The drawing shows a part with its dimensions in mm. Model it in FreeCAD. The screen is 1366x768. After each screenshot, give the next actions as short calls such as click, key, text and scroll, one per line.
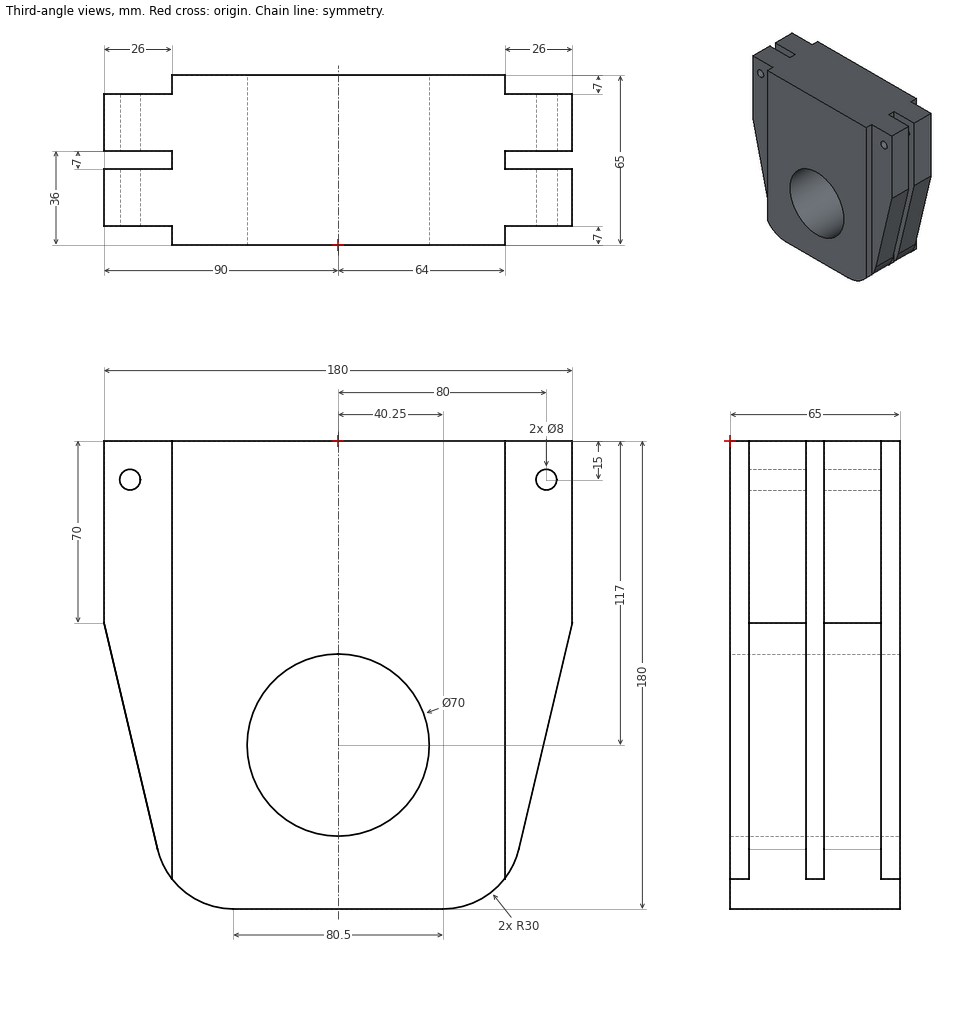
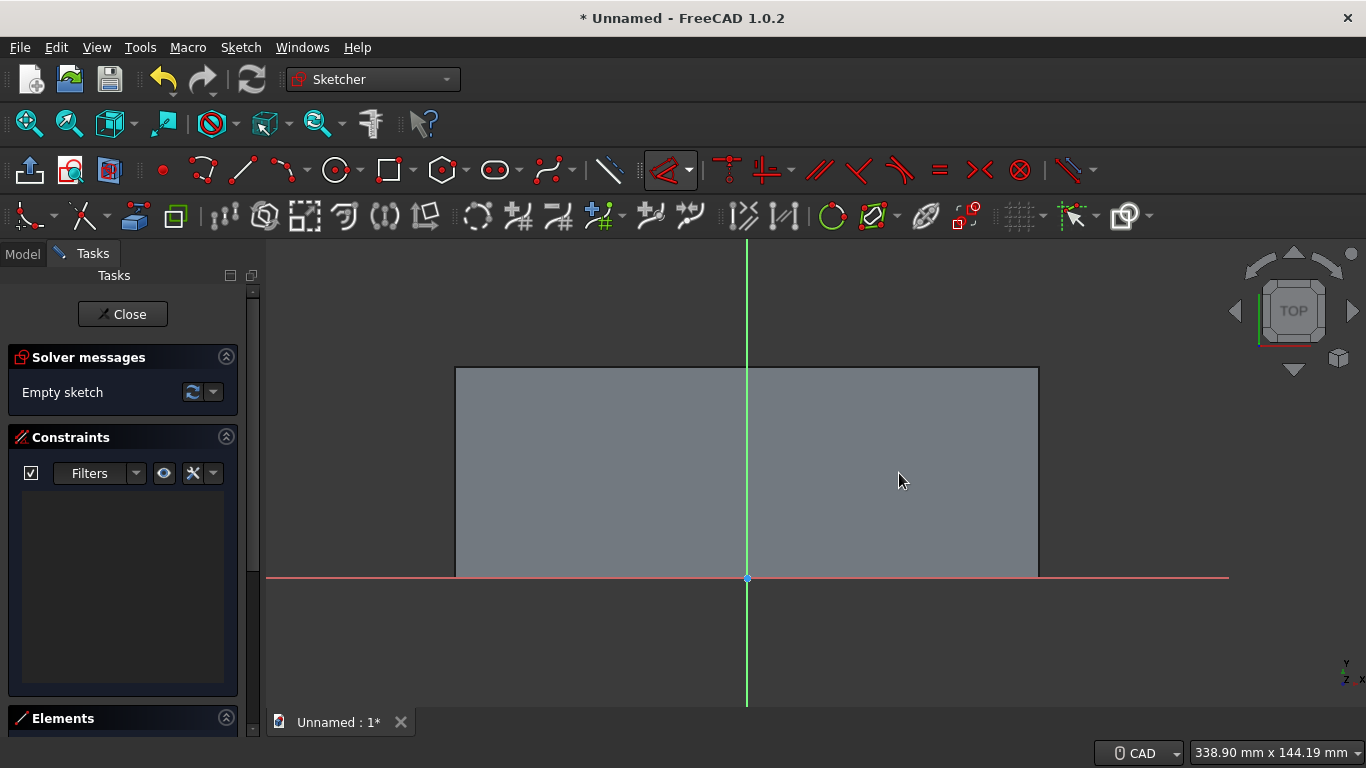
click(390, 170)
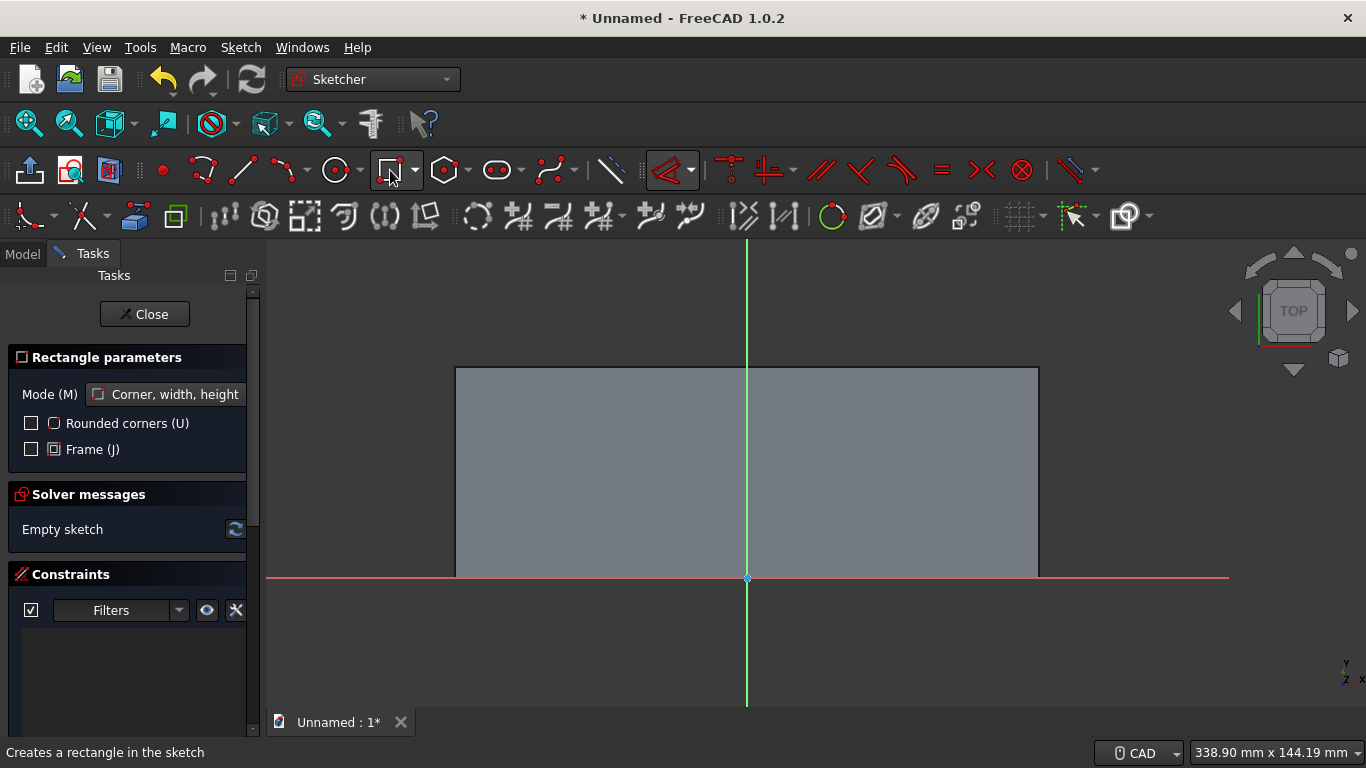
click(955, 555)
click(1039, 578)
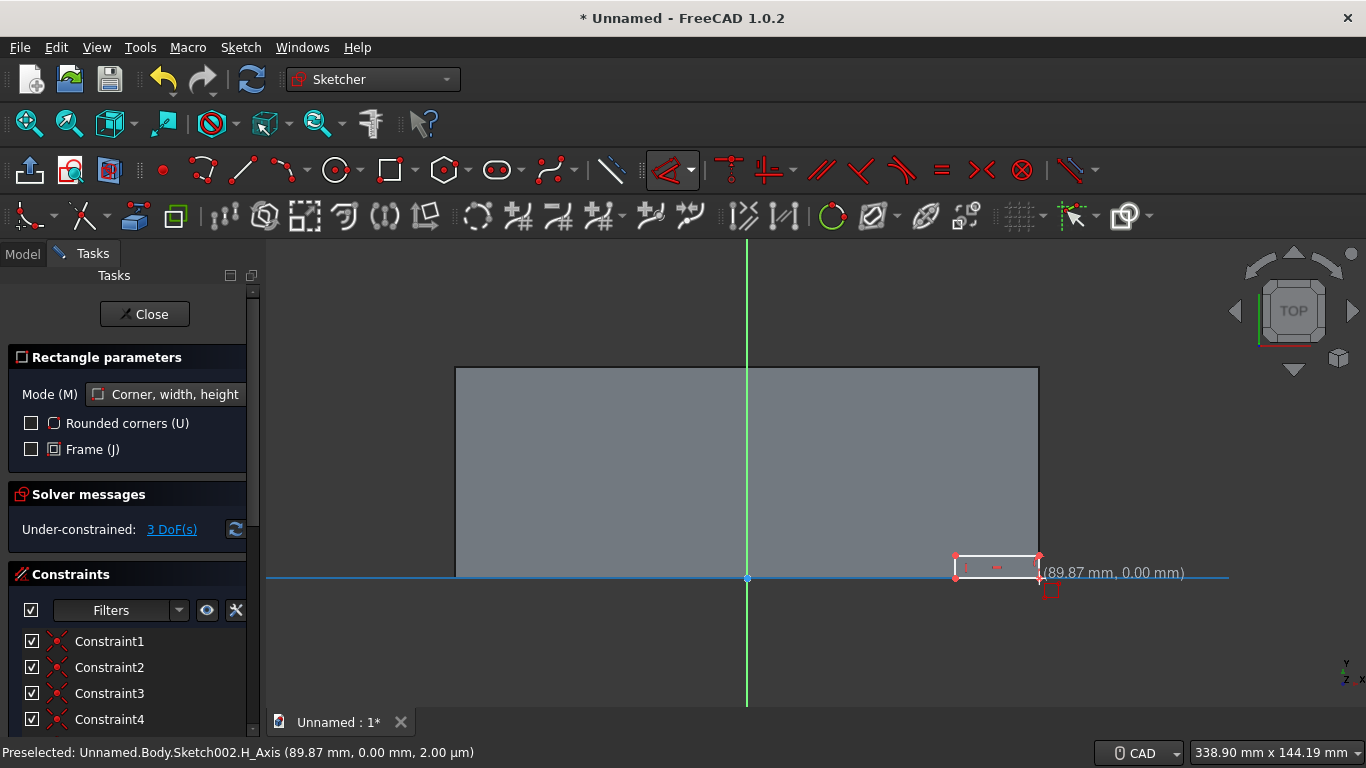
click(955, 367)
move(1039, 390)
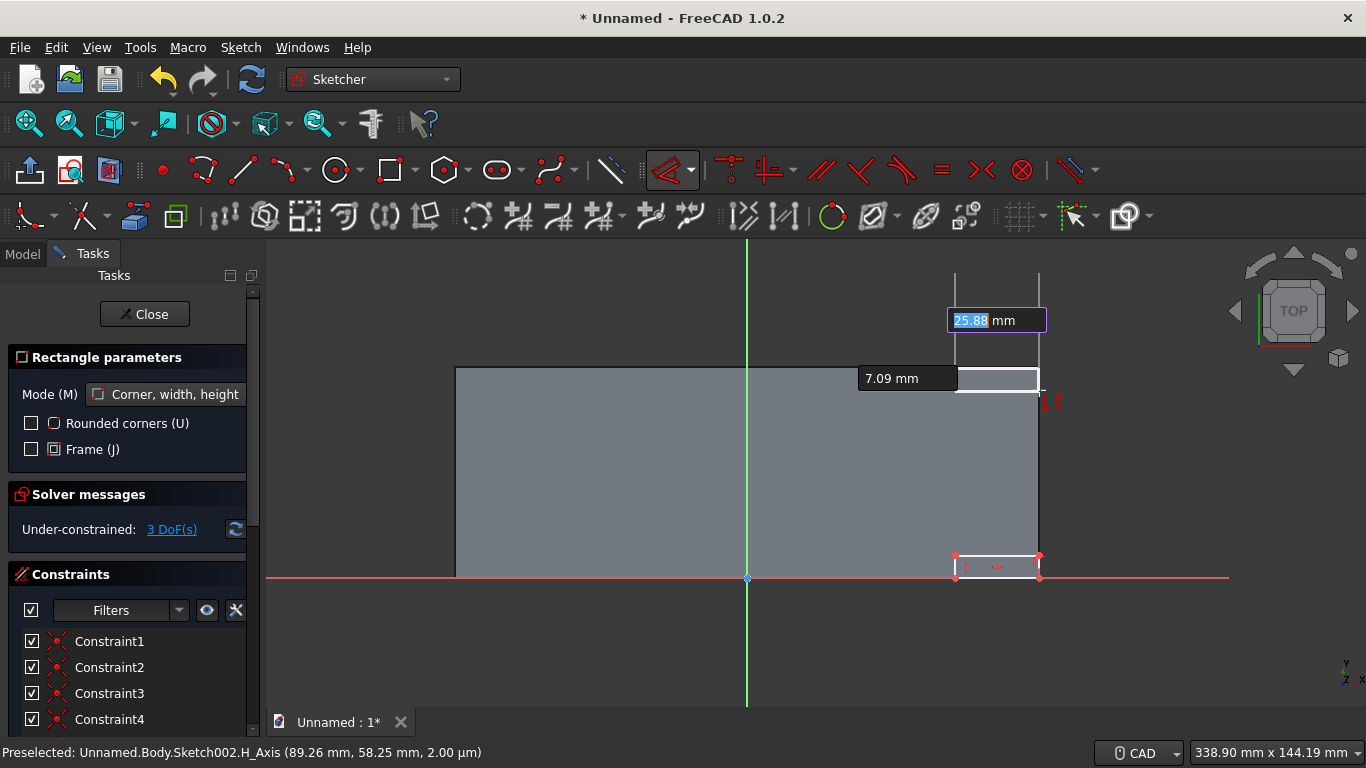
text(26)
key(Tab)
text(7)
key(Return)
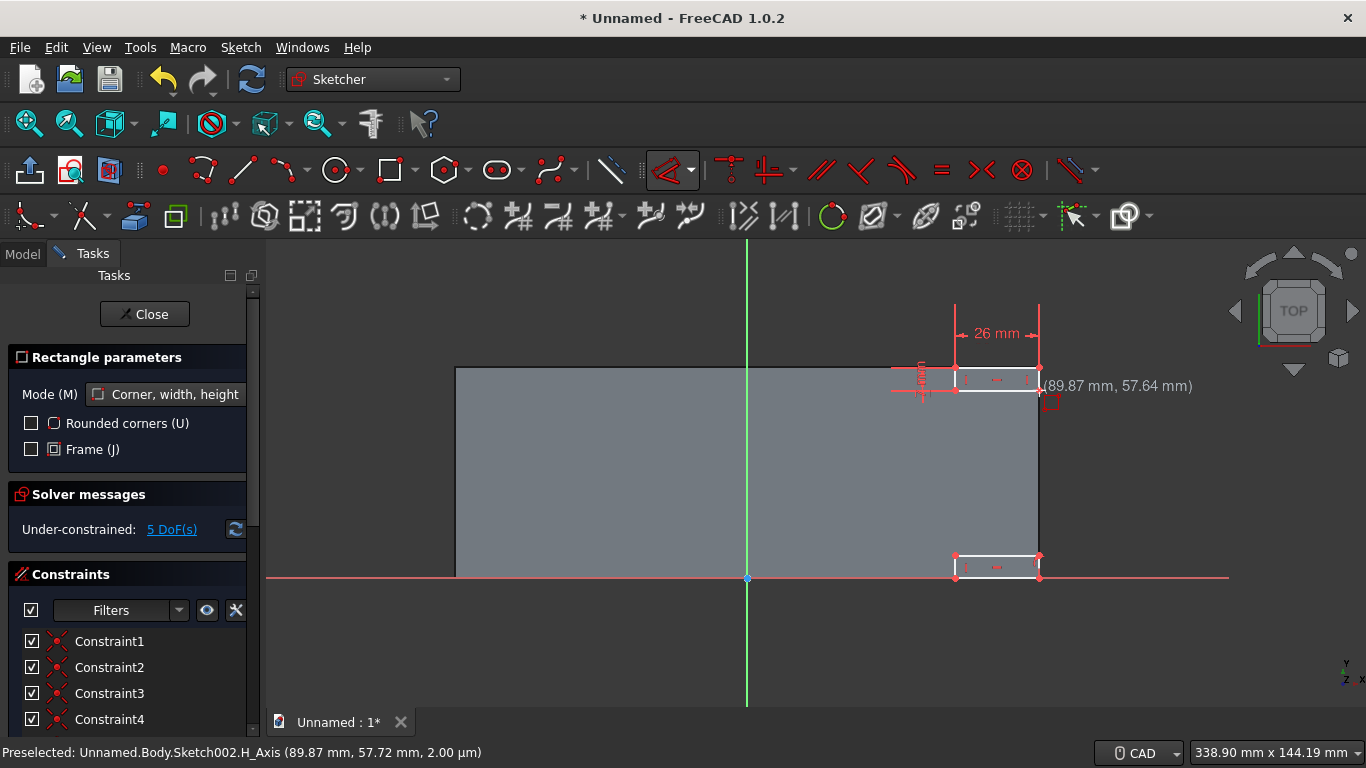
click(455, 367)
move(540, 390)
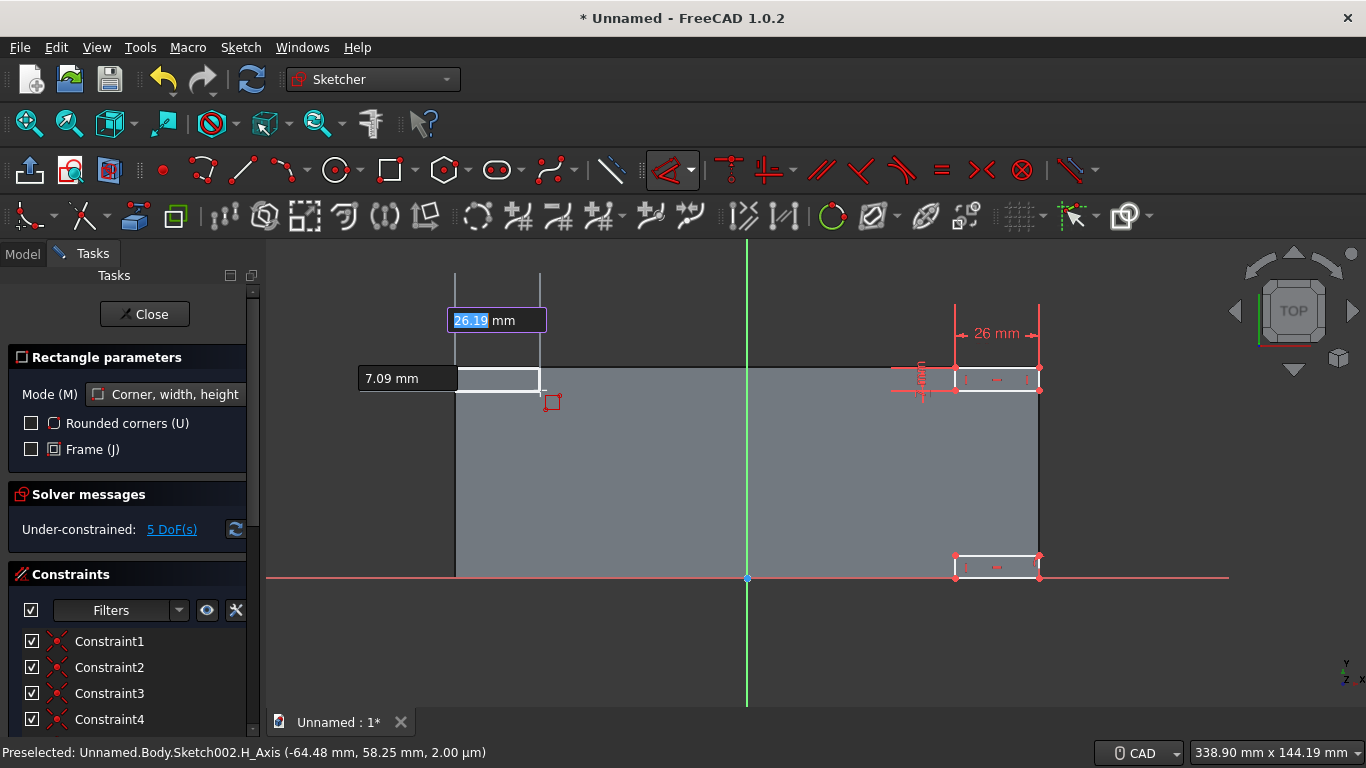
text(26)
key(Tab)
text(7)
key(Return)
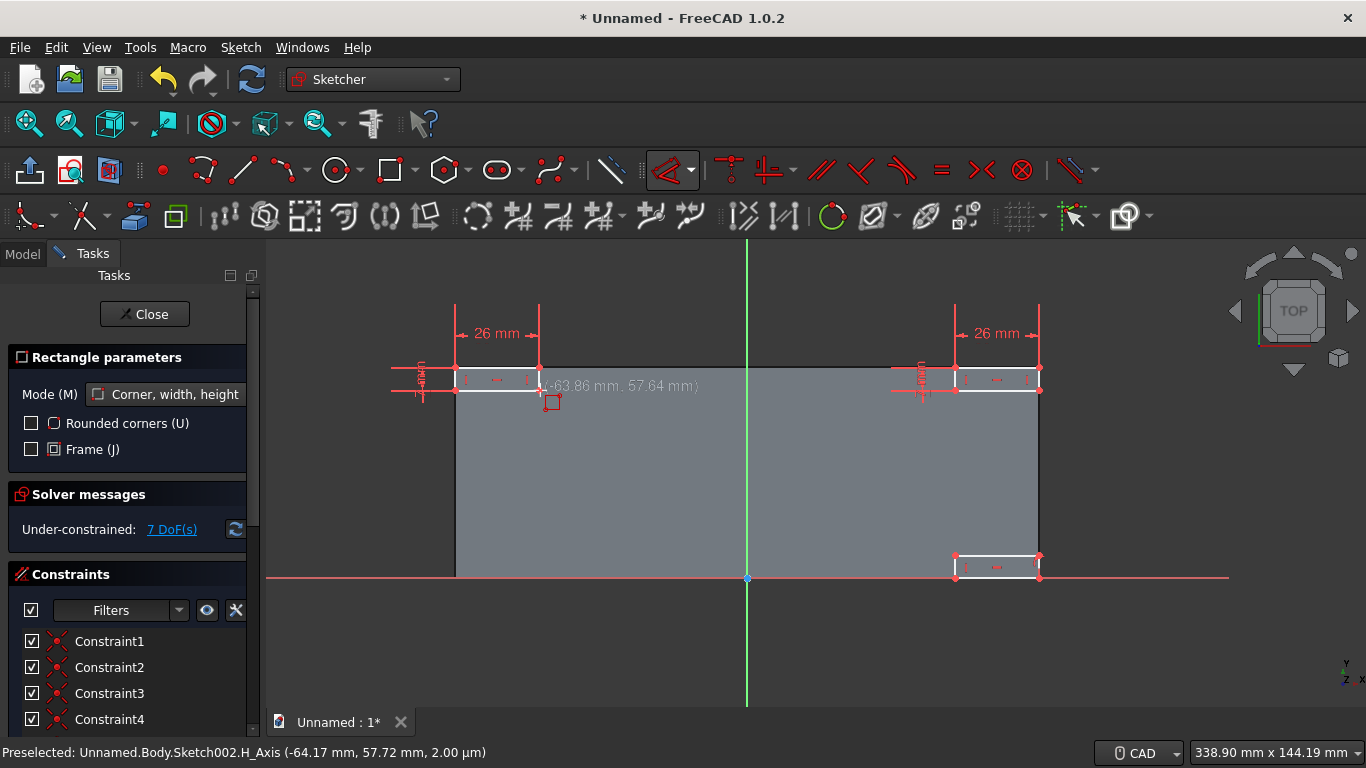
click(455, 555)
click(540, 578)
key(Escape)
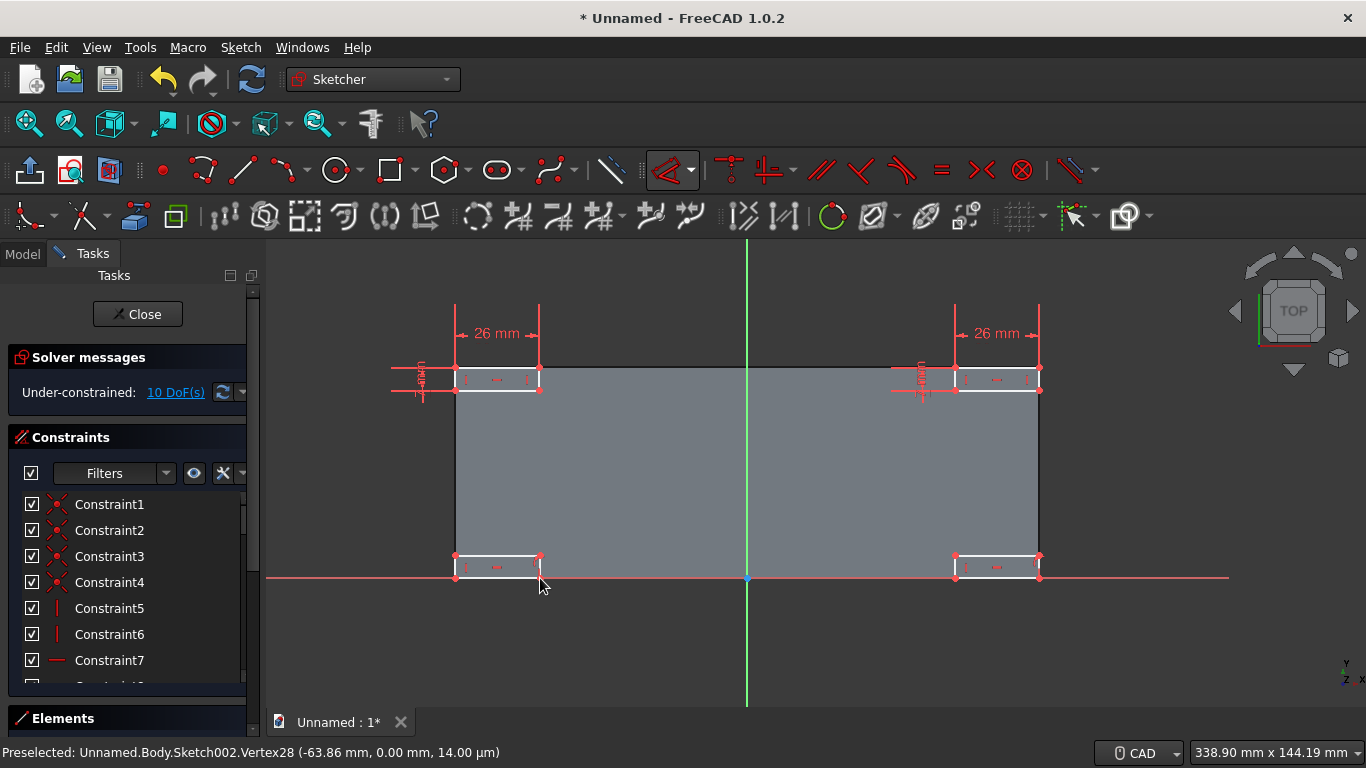
click(1039, 368)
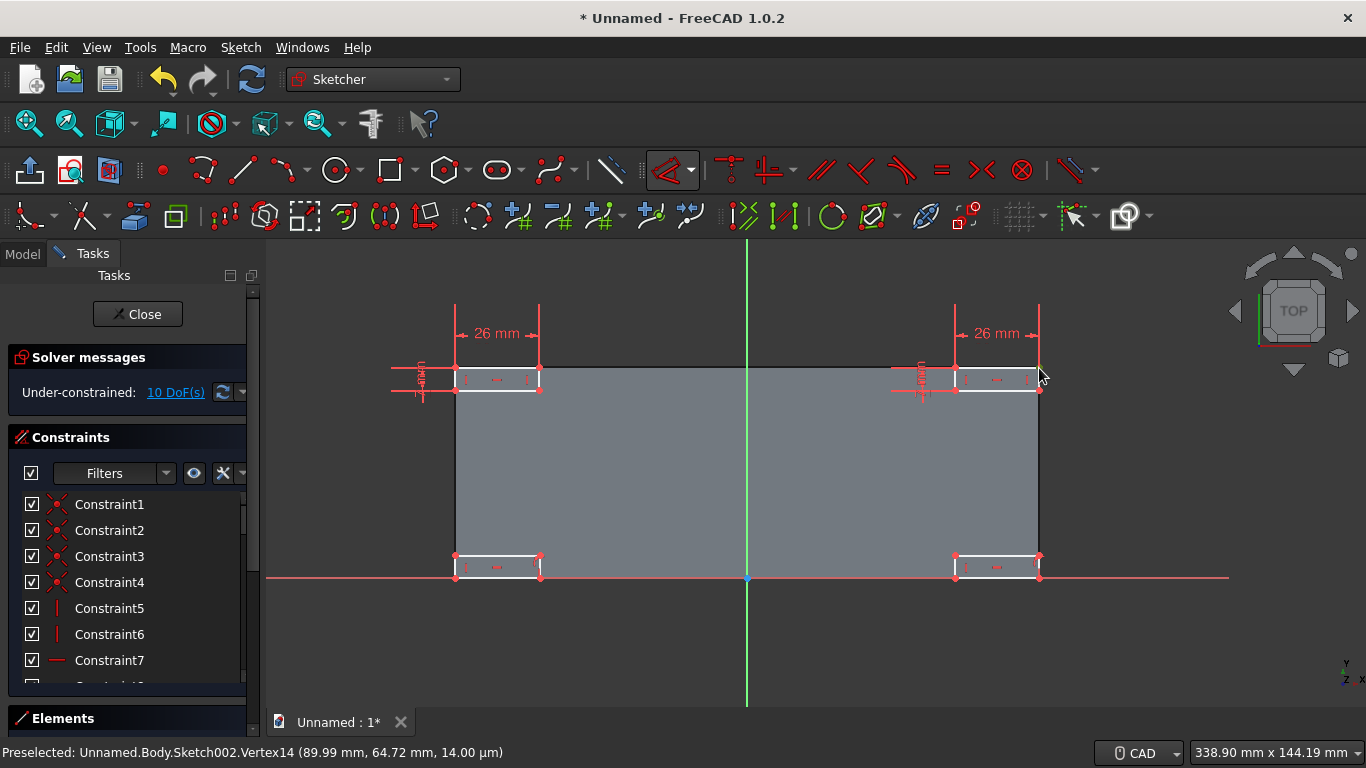
click(455, 368)